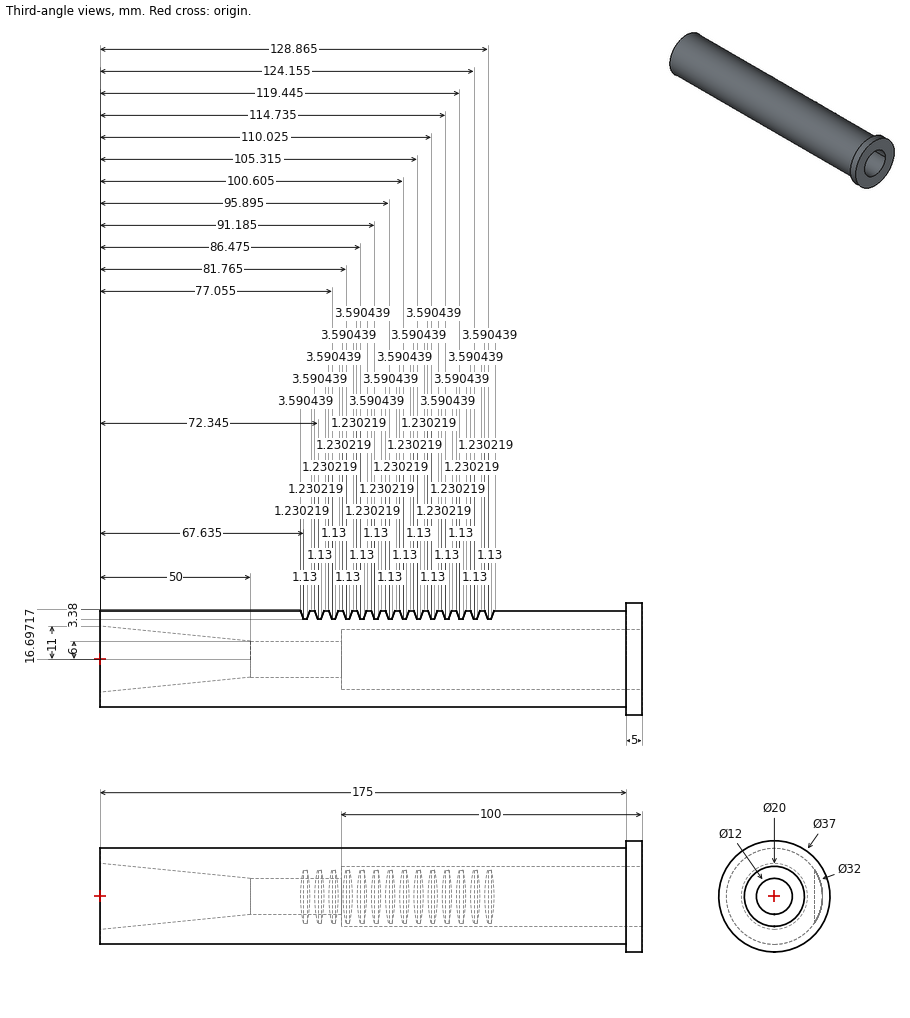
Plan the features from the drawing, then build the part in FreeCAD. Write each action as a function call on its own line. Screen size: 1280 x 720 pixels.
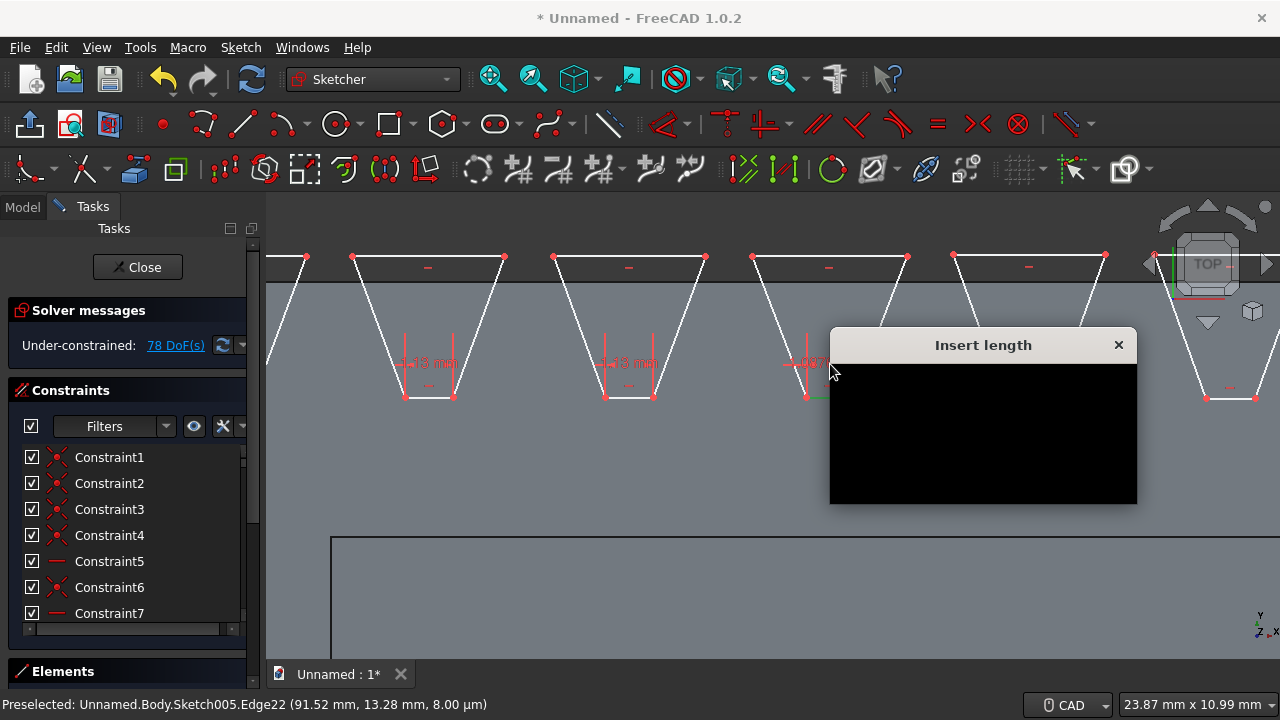
text(1.13)
key(Return)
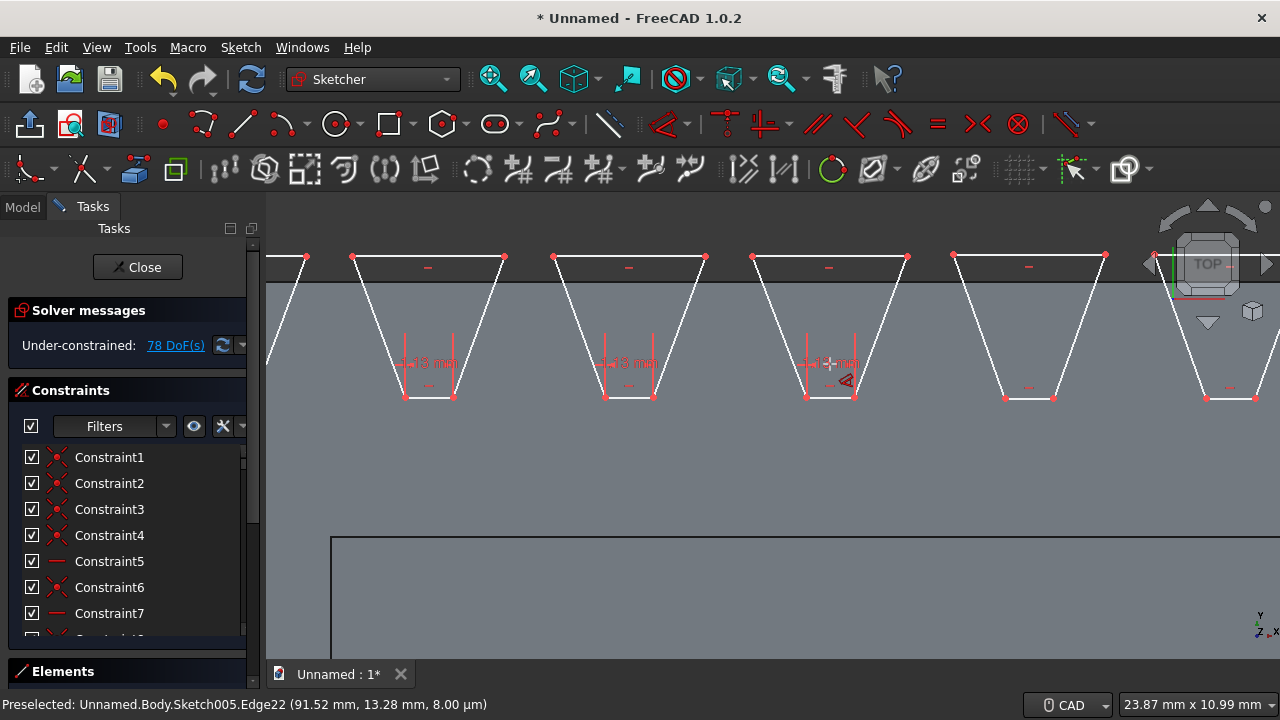
click(1020, 399)
click(1029, 365)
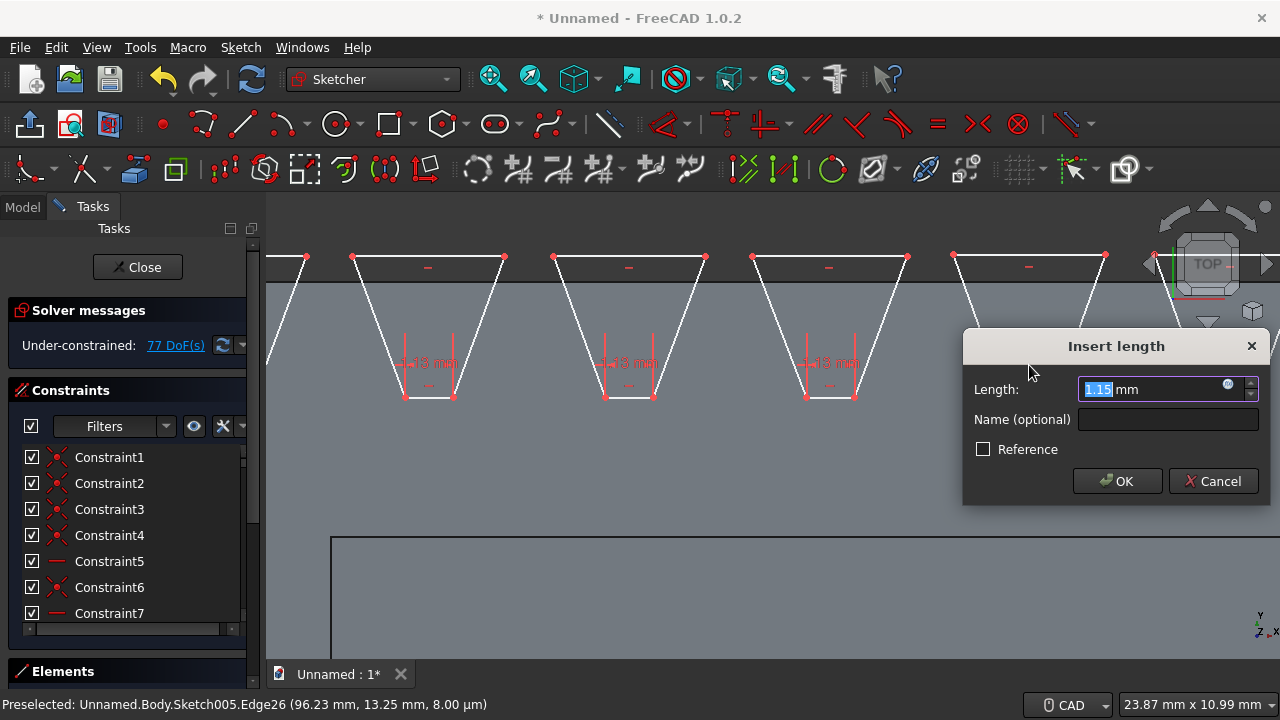
text(1.13)
key(Return)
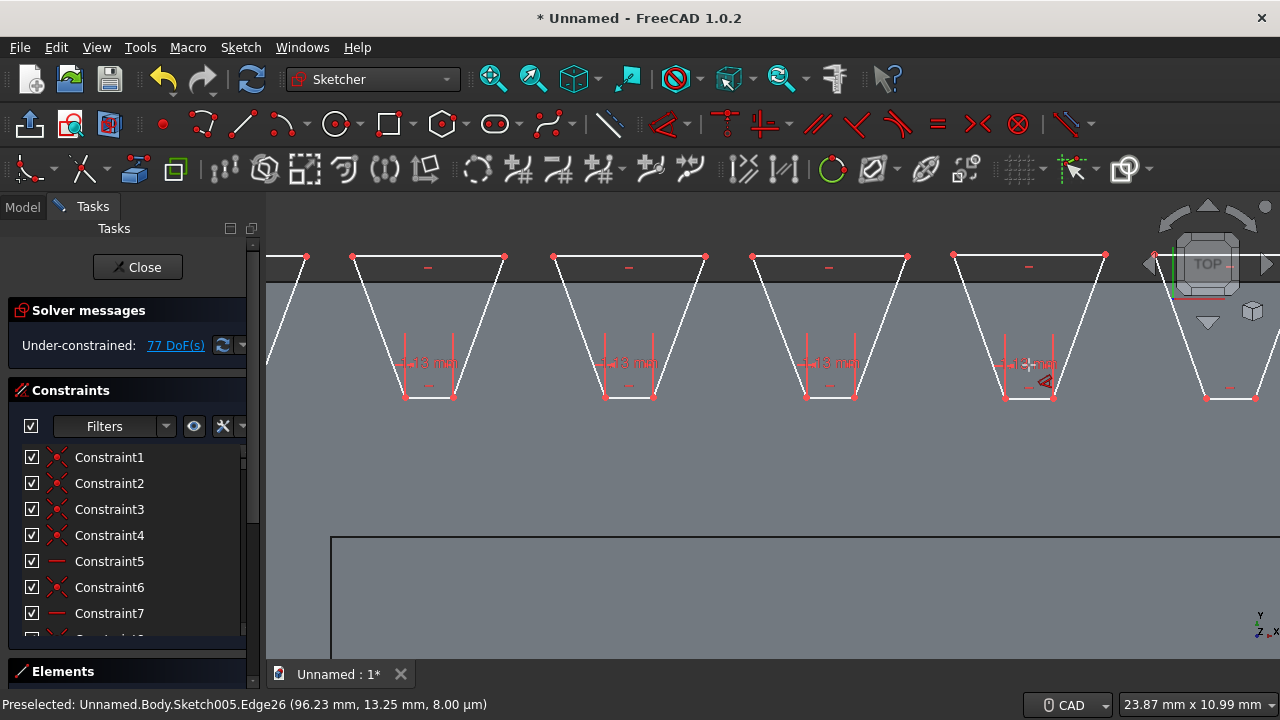
scroll(827, 403, down, 11)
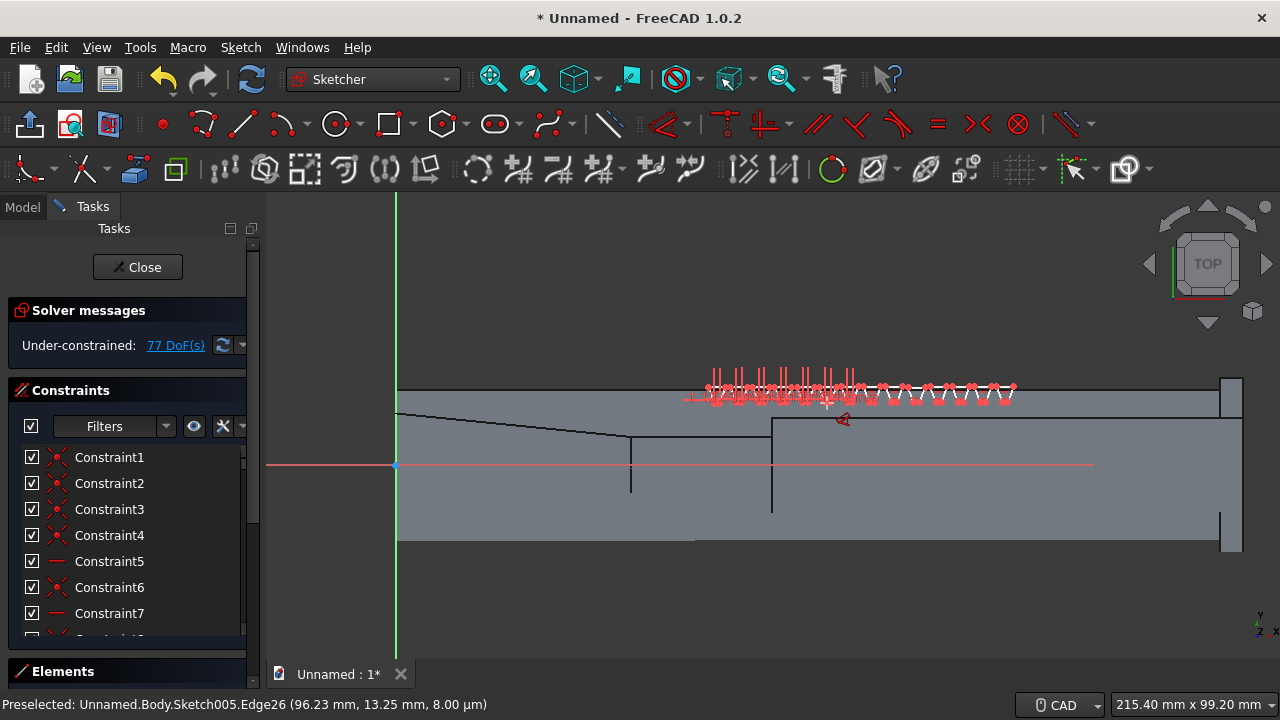
scroll(871, 403, up, 11)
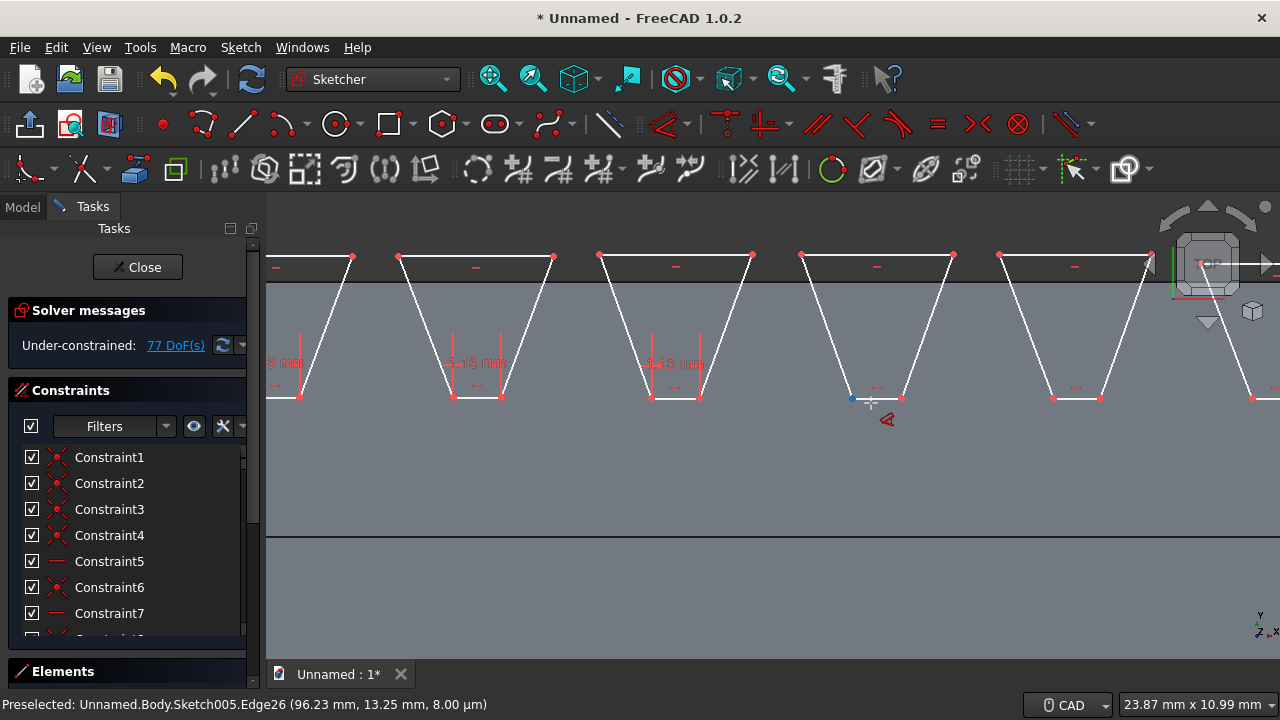
click(867, 399)
click(877, 365)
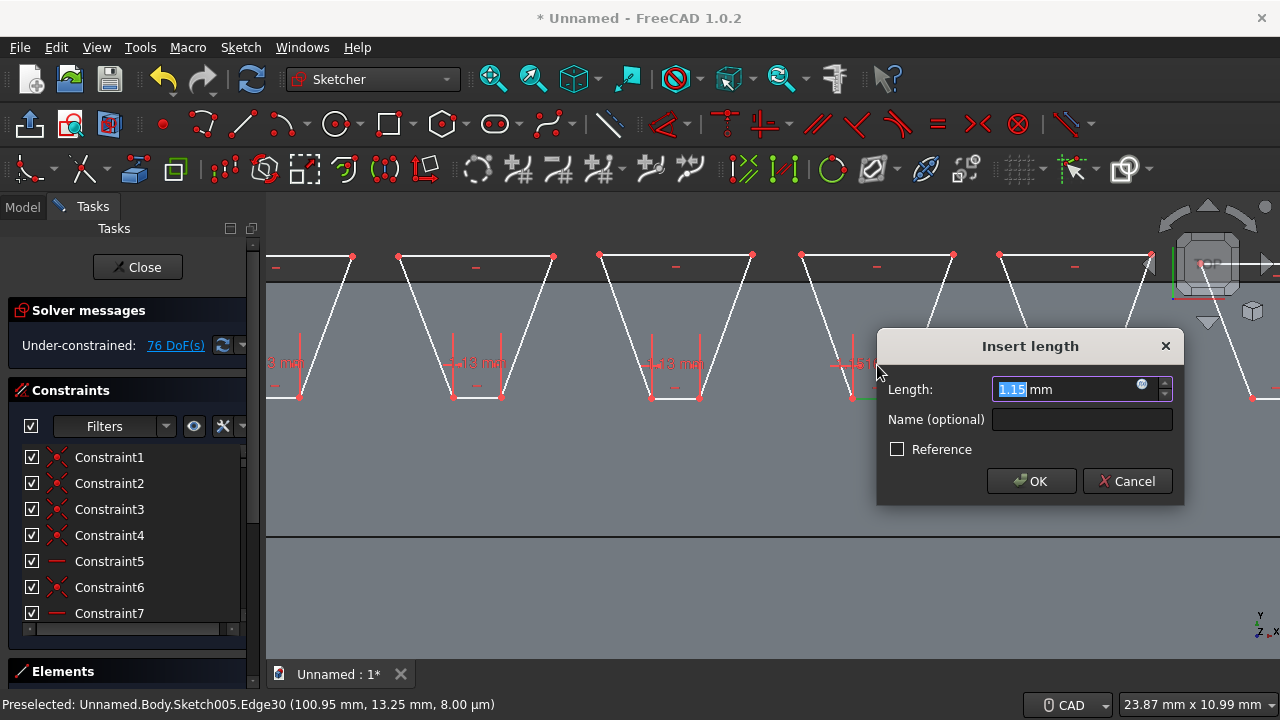
text(1.13)
key(Return)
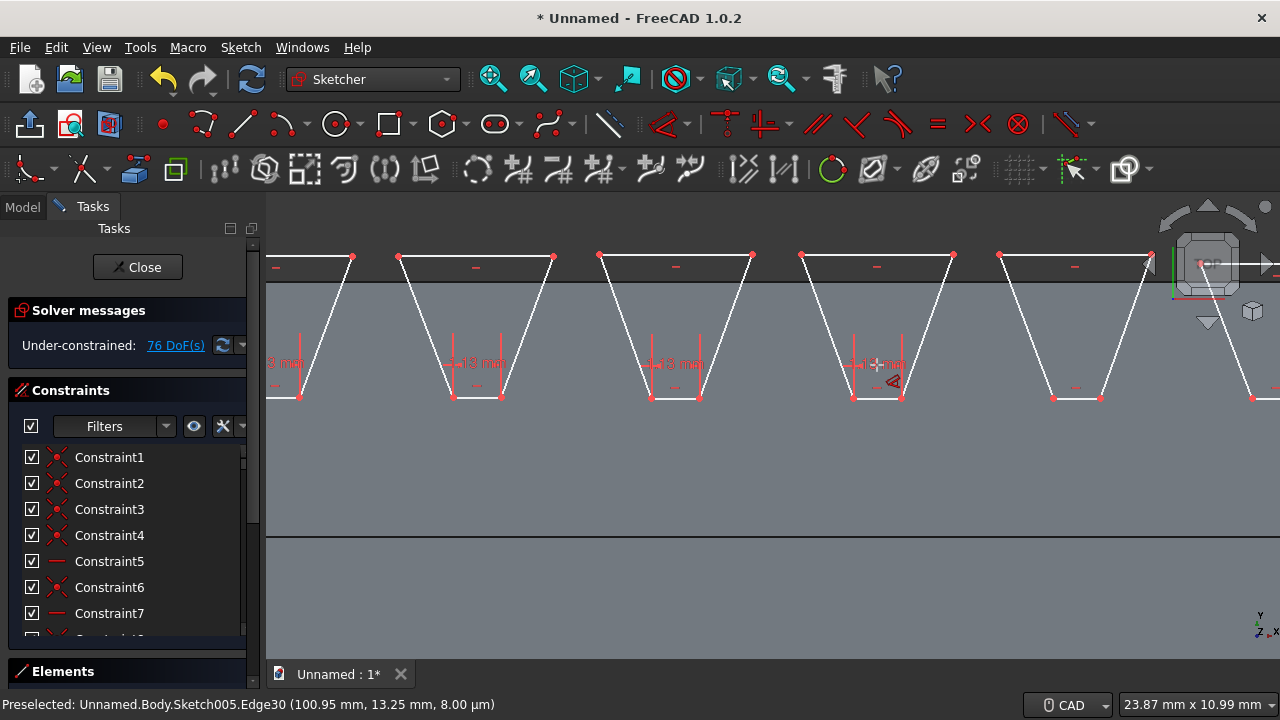
click(1068, 399)
click(1077, 365)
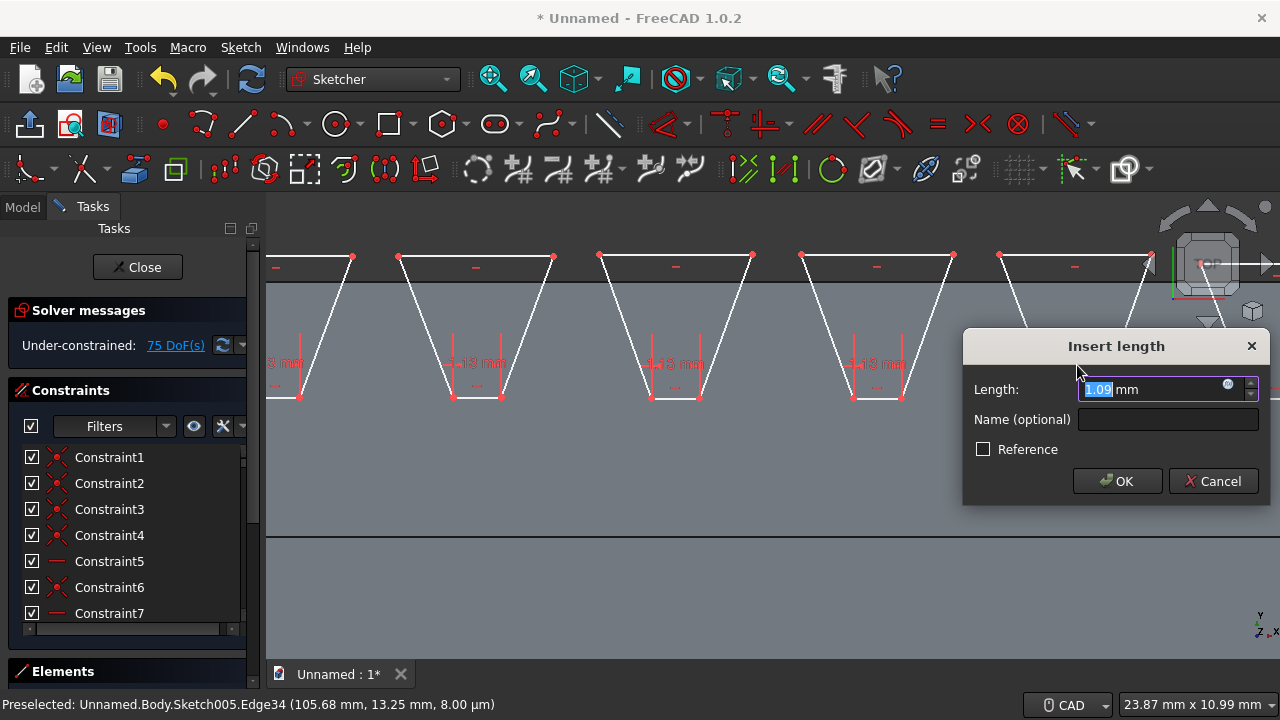
text(1.13)
key(Return)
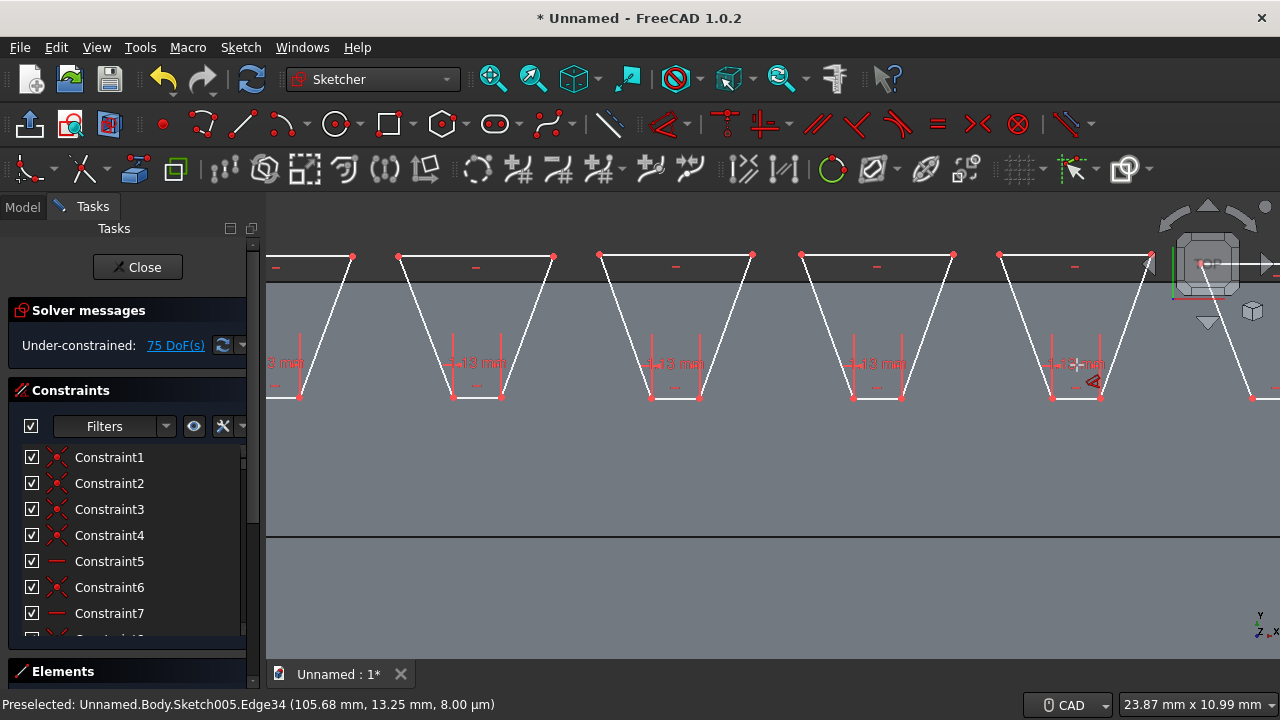
scroll(871, 403, down, 11)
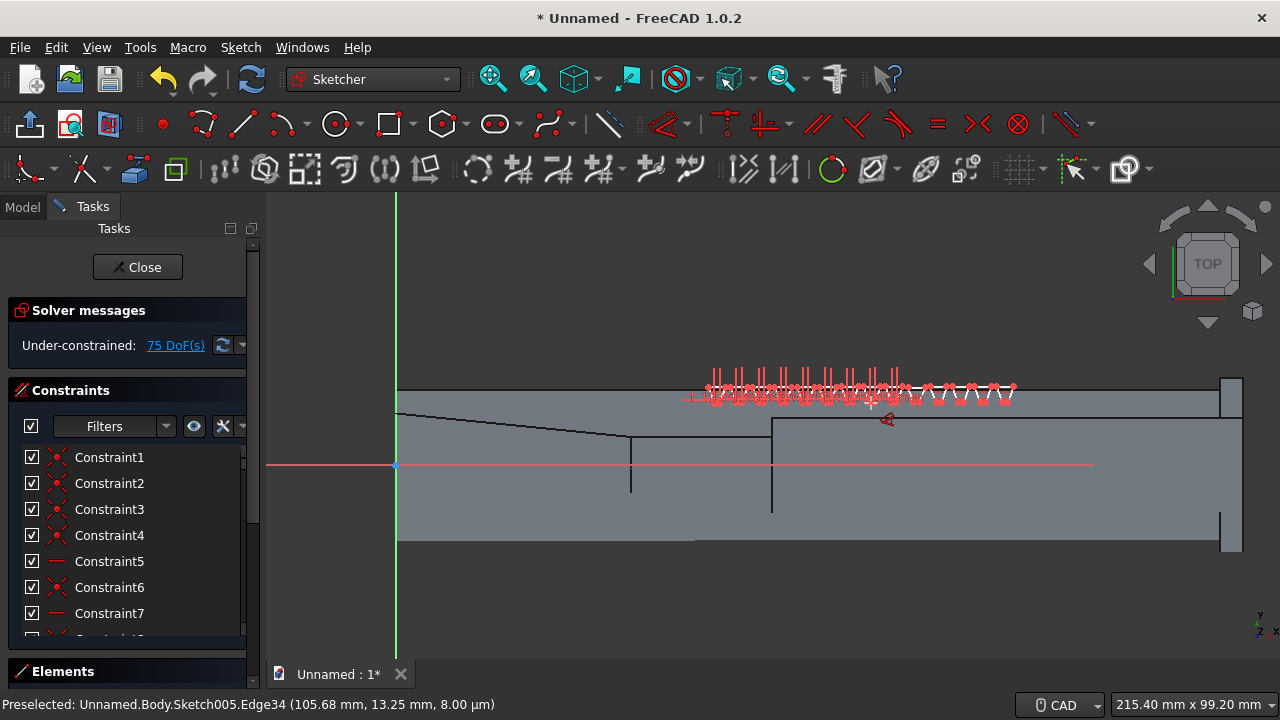
scroll(915, 403, up, 11)